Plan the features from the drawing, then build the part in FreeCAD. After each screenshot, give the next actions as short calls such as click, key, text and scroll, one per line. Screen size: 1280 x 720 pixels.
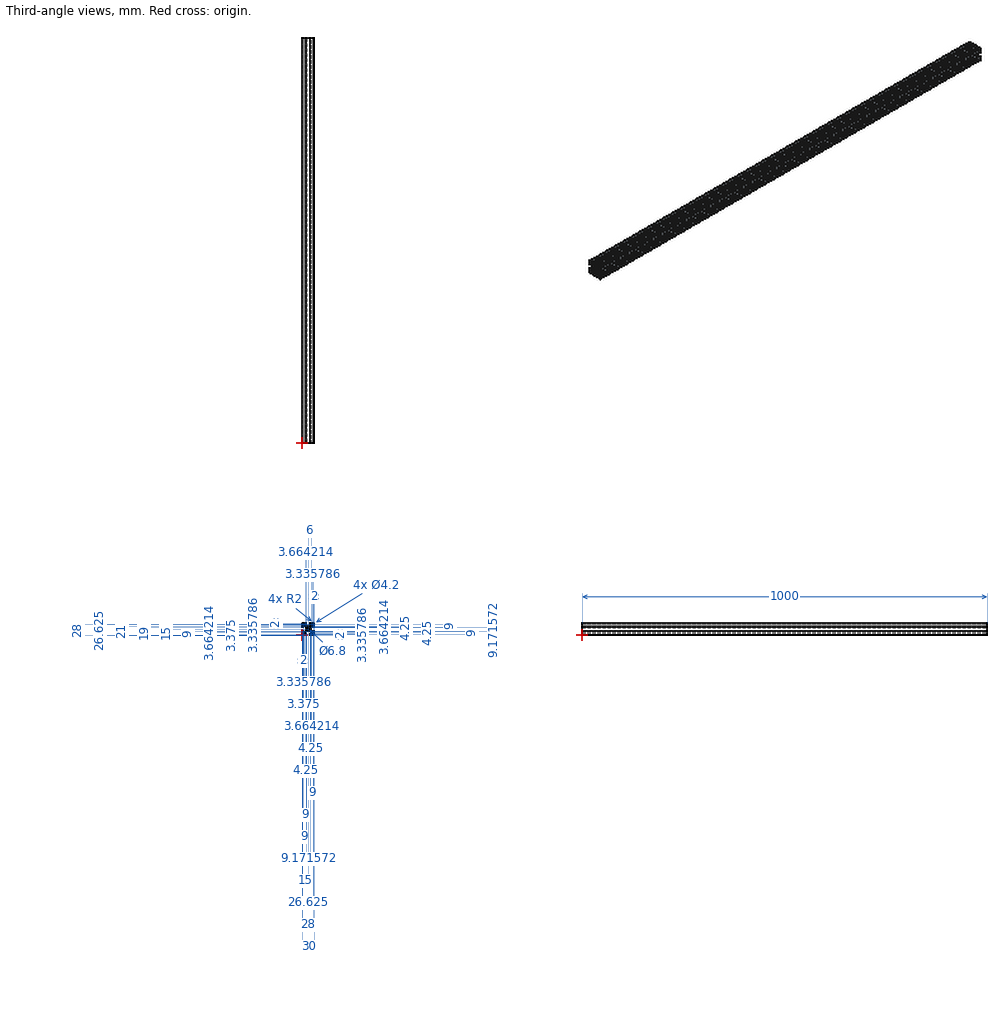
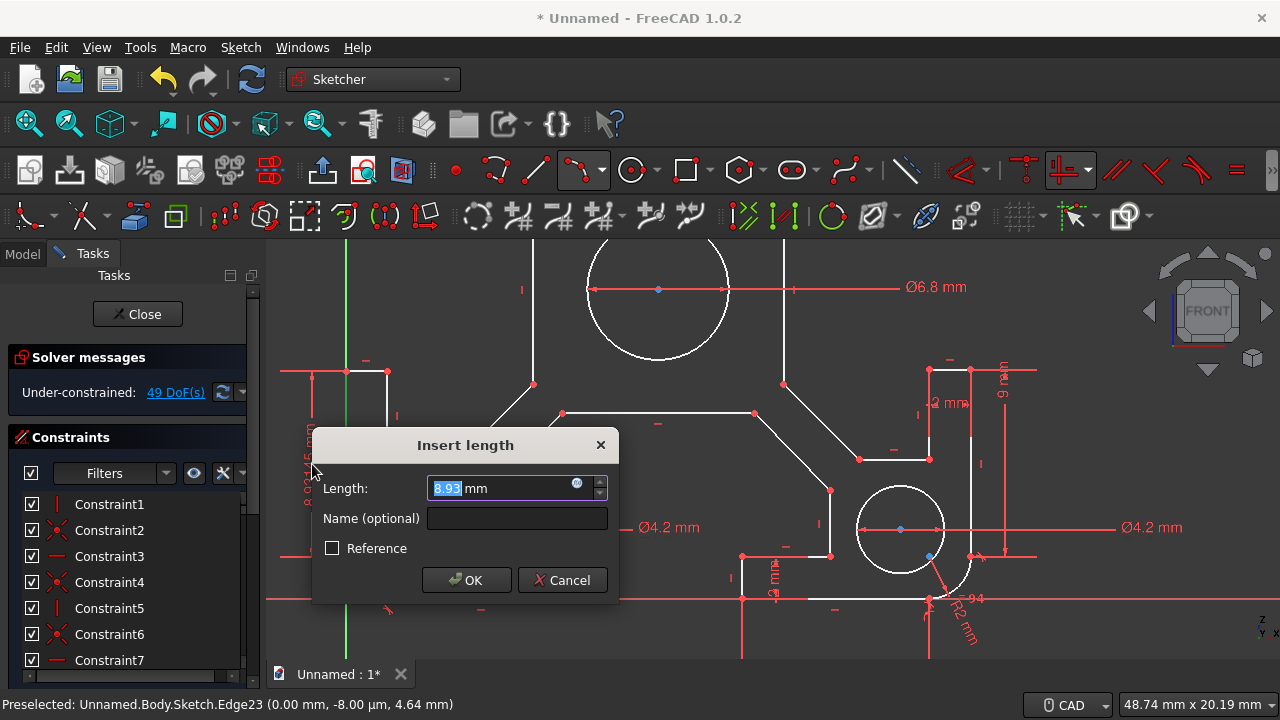
text(9)
key(Return)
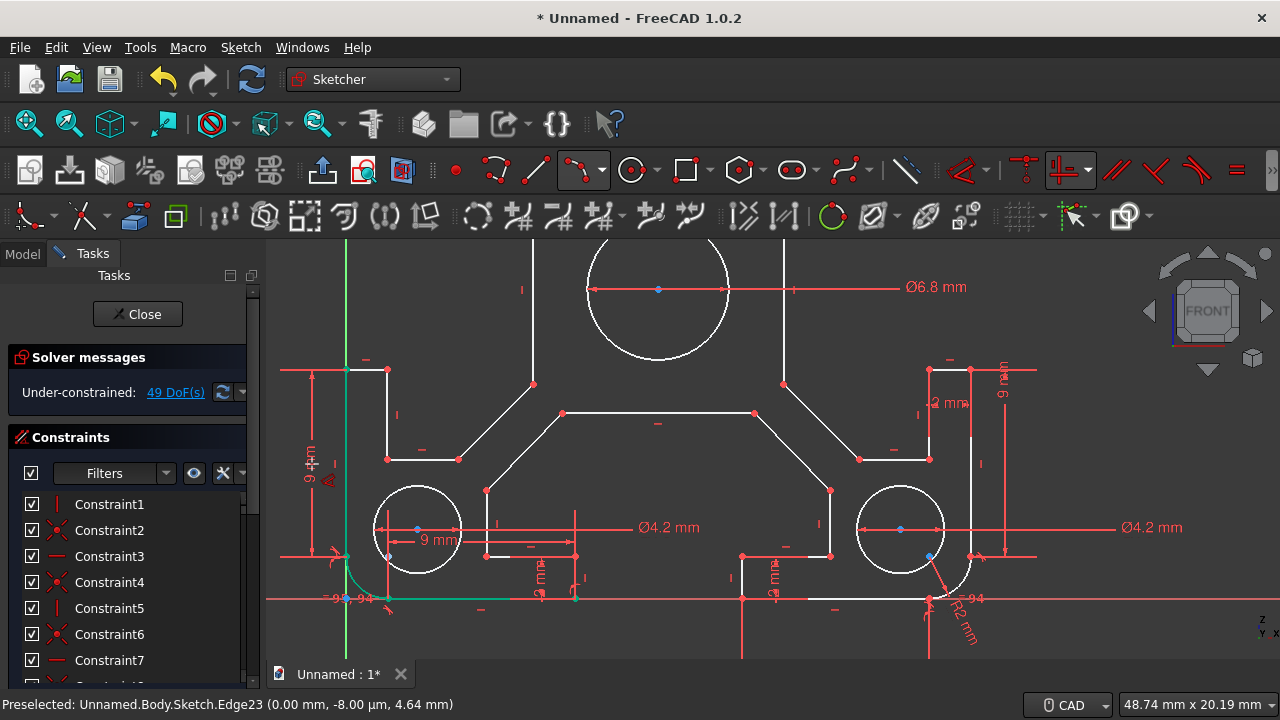
click(359, 370)
click(367, 404)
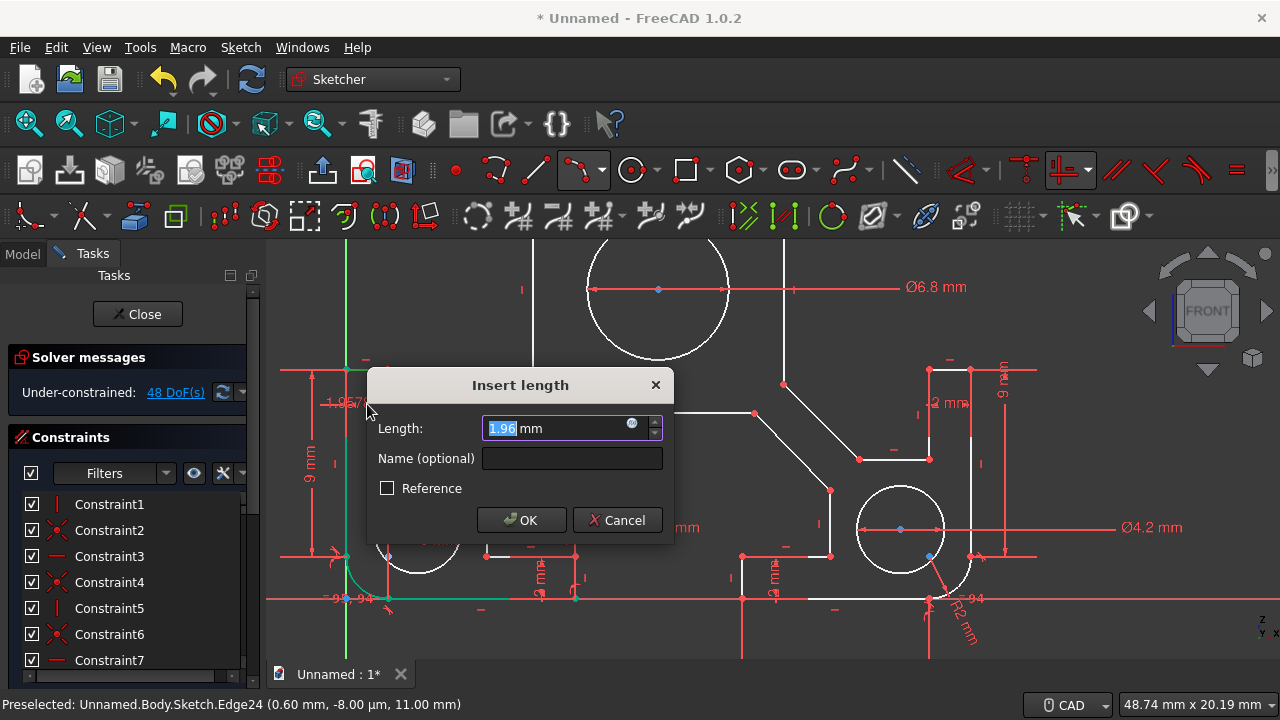
text(2)
key(Return)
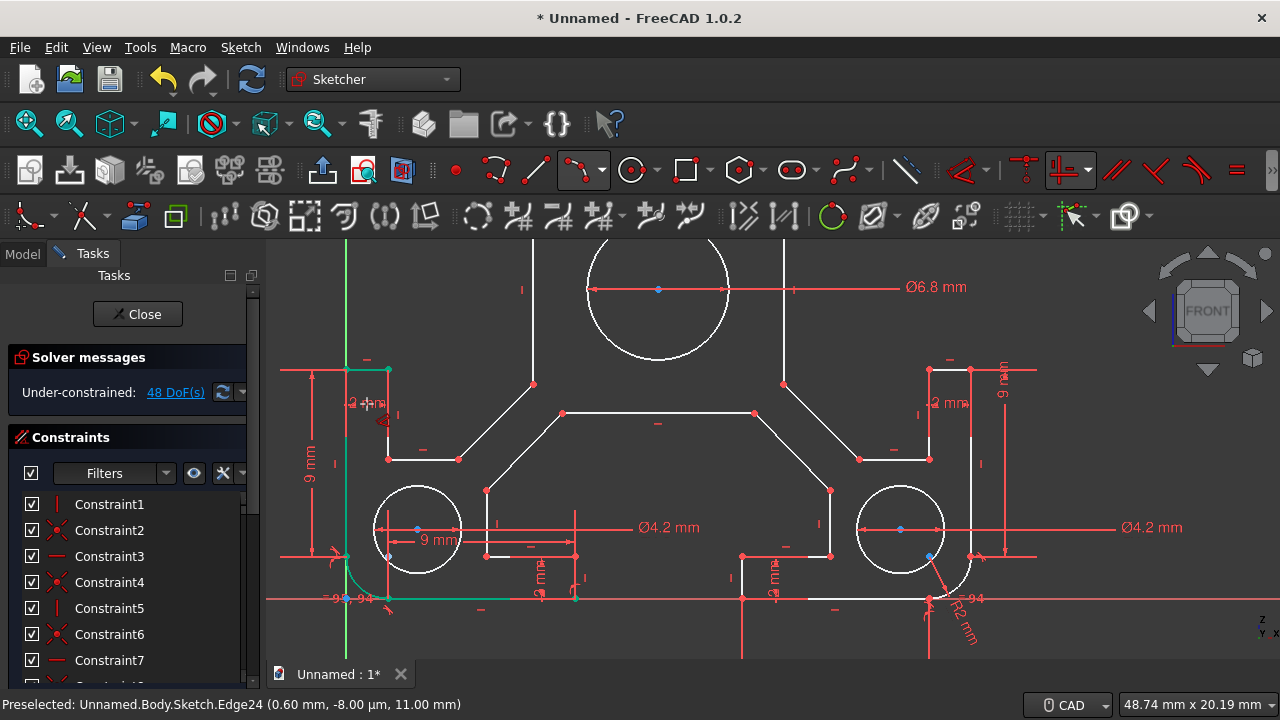
scroll(742, 582, down, 4)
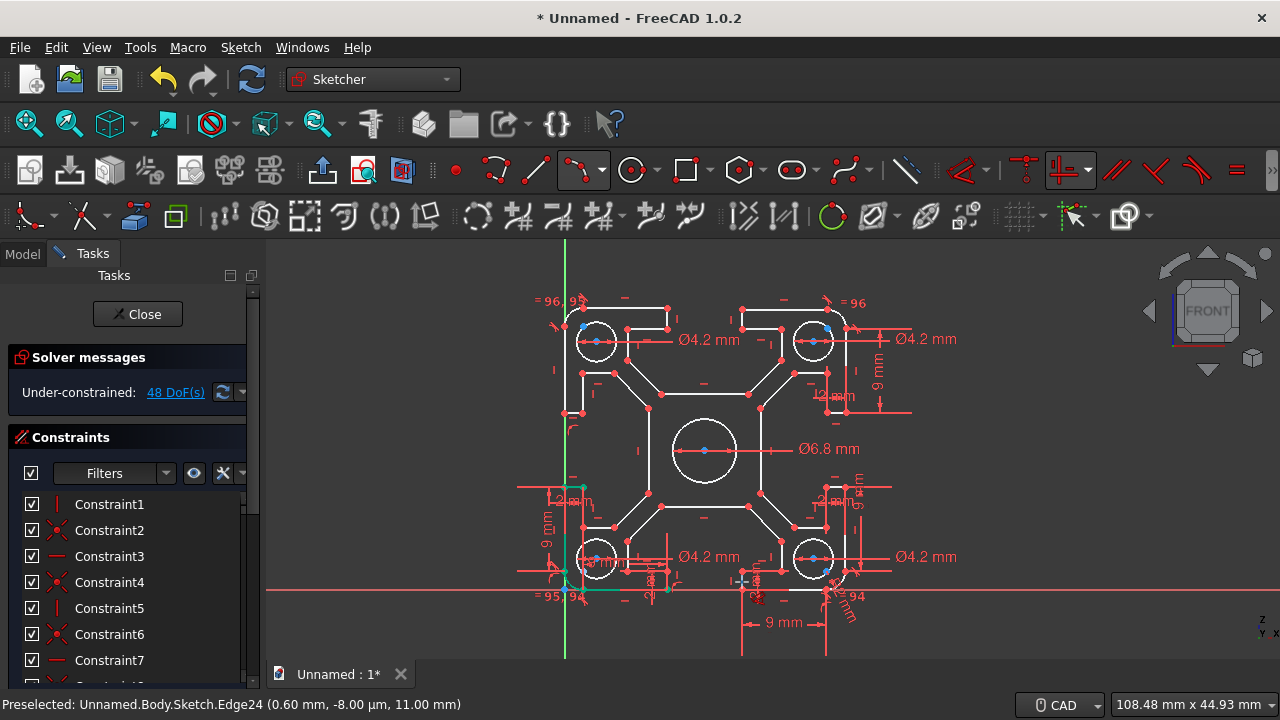
scroll(577, 413, up, 5)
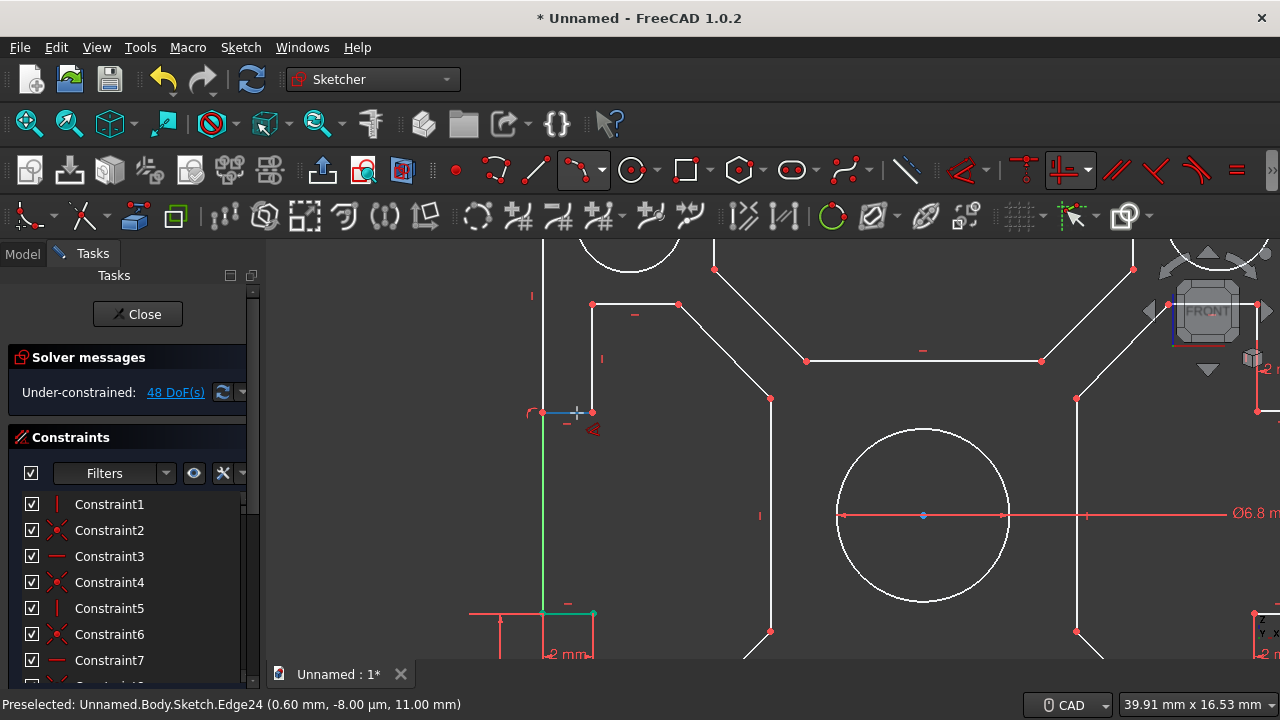
click(577, 413)
click(567, 379)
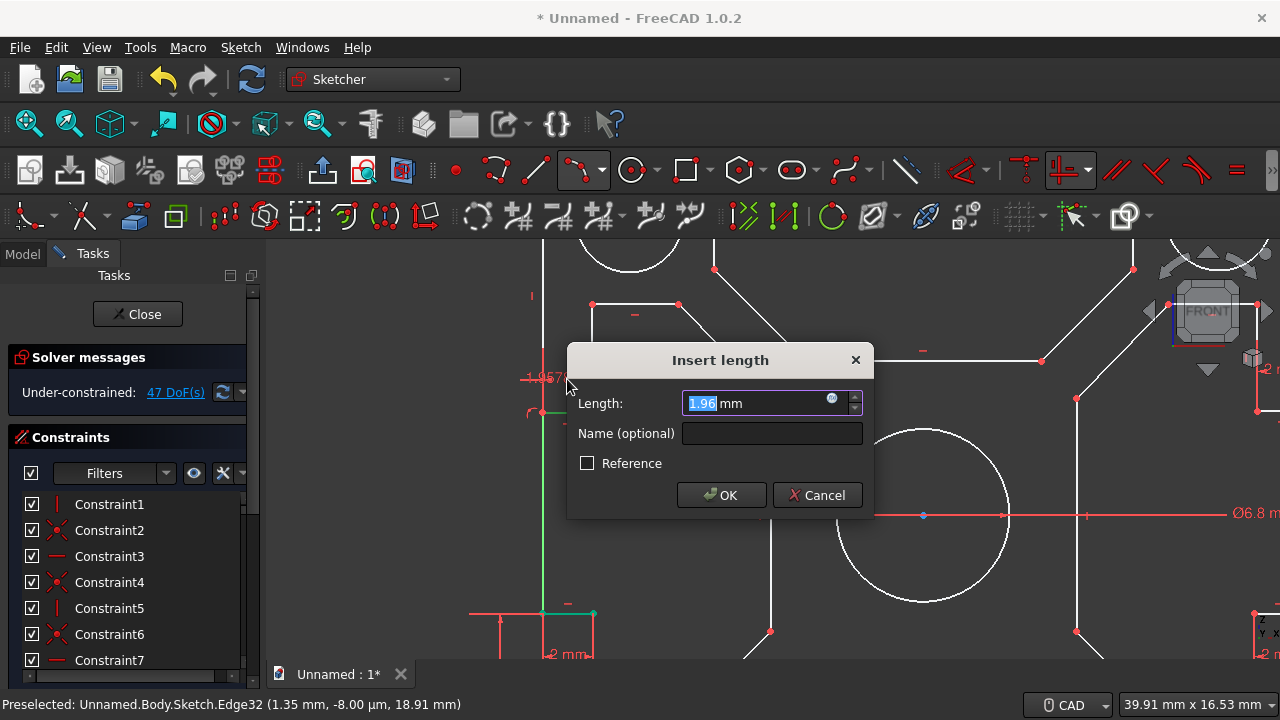
text(2)
key(Return)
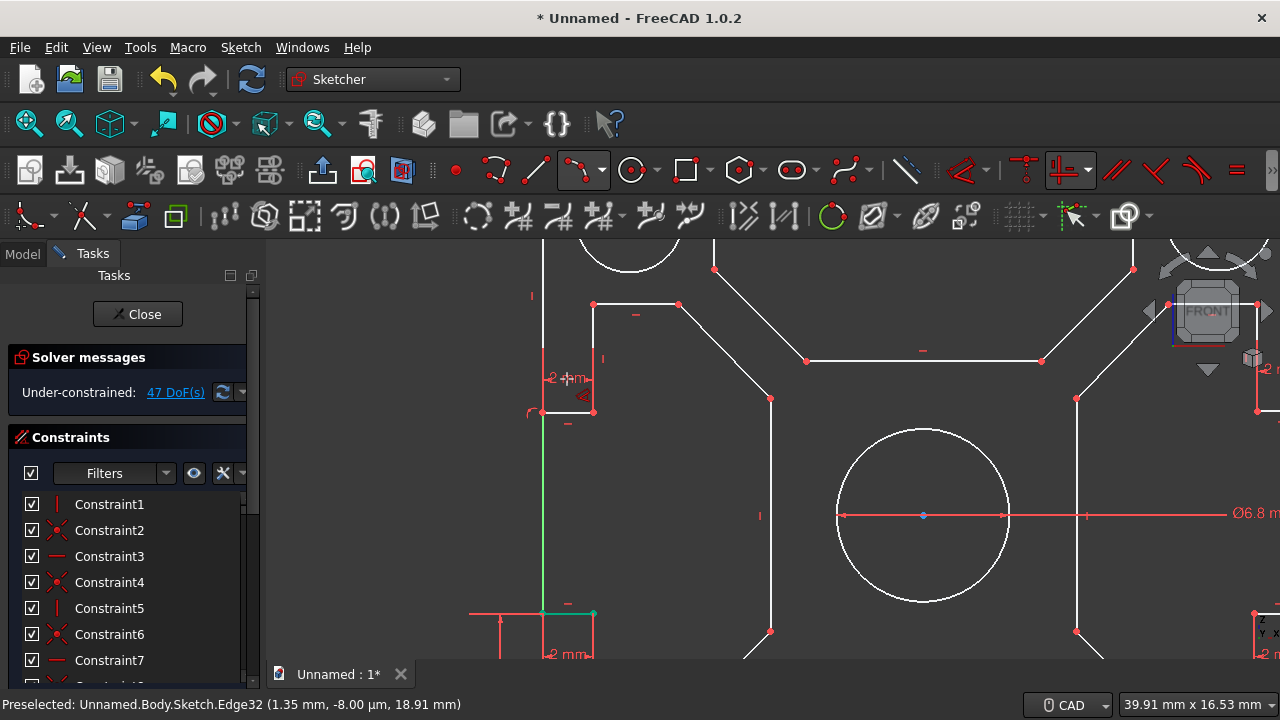
click(543, 342)
click(509, 340)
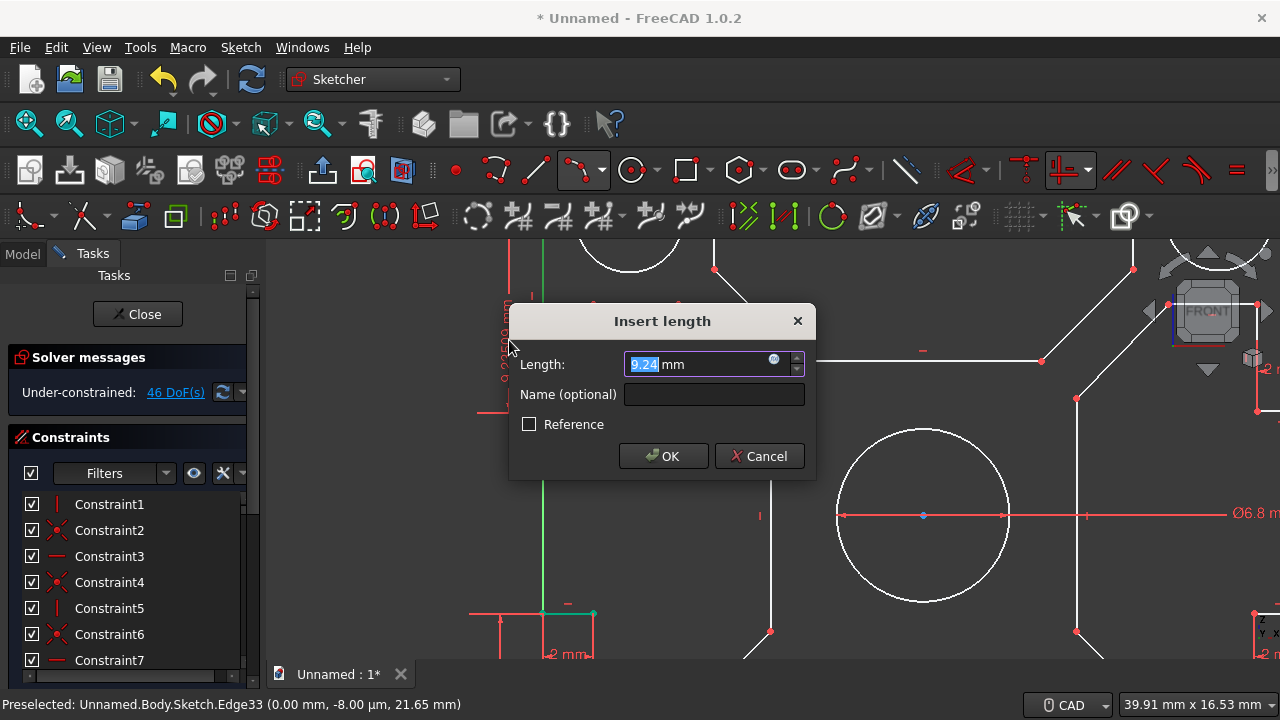
text(9)
key(Return)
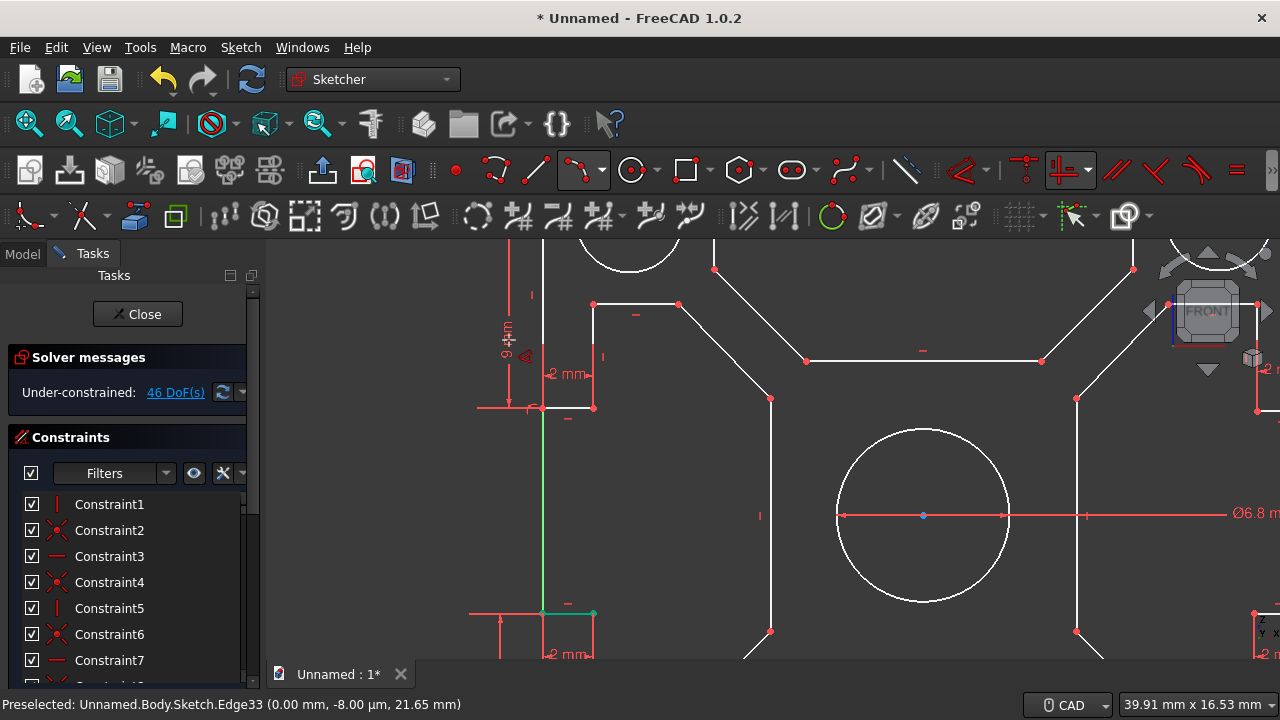
scroll(577, 412, down, 5)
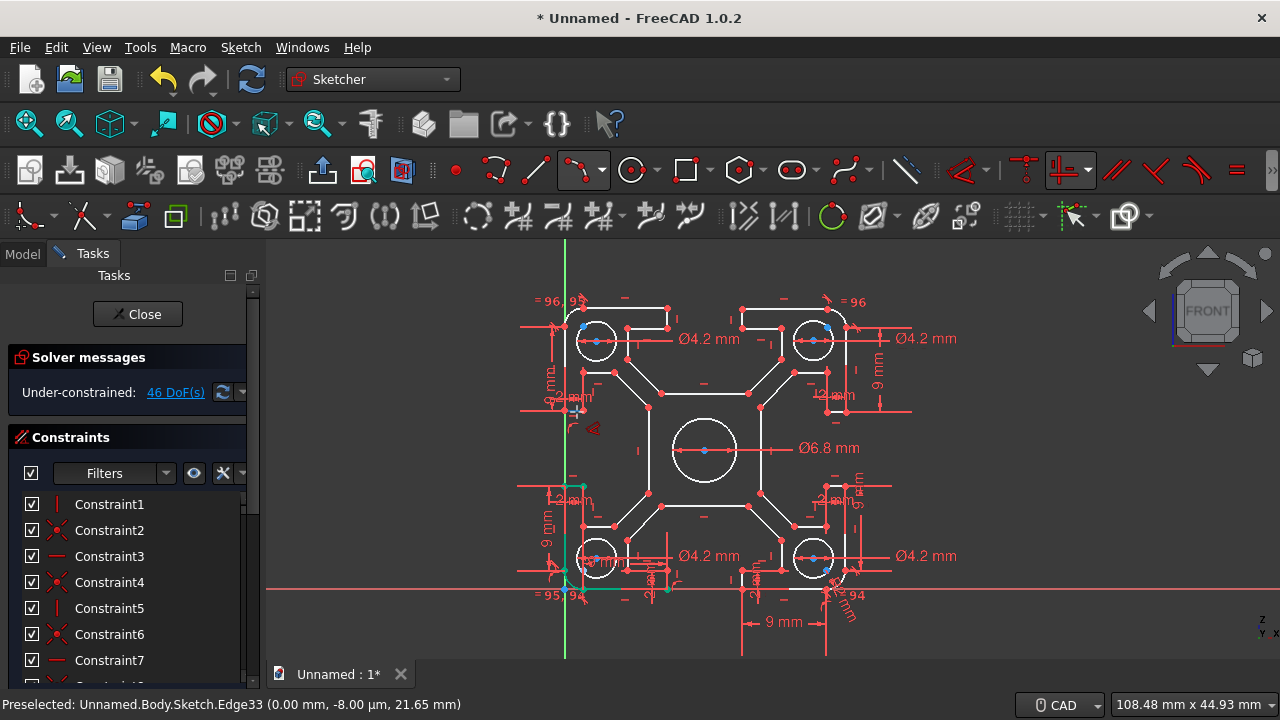
click(609, 308)
click(625, 274)